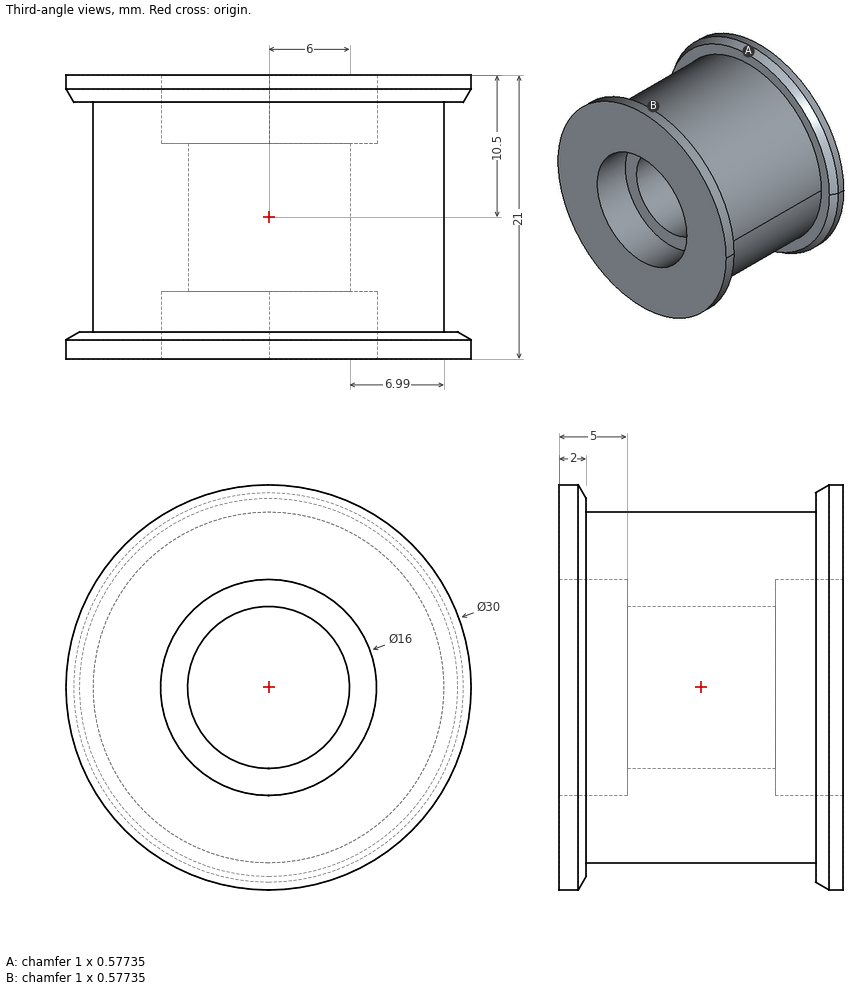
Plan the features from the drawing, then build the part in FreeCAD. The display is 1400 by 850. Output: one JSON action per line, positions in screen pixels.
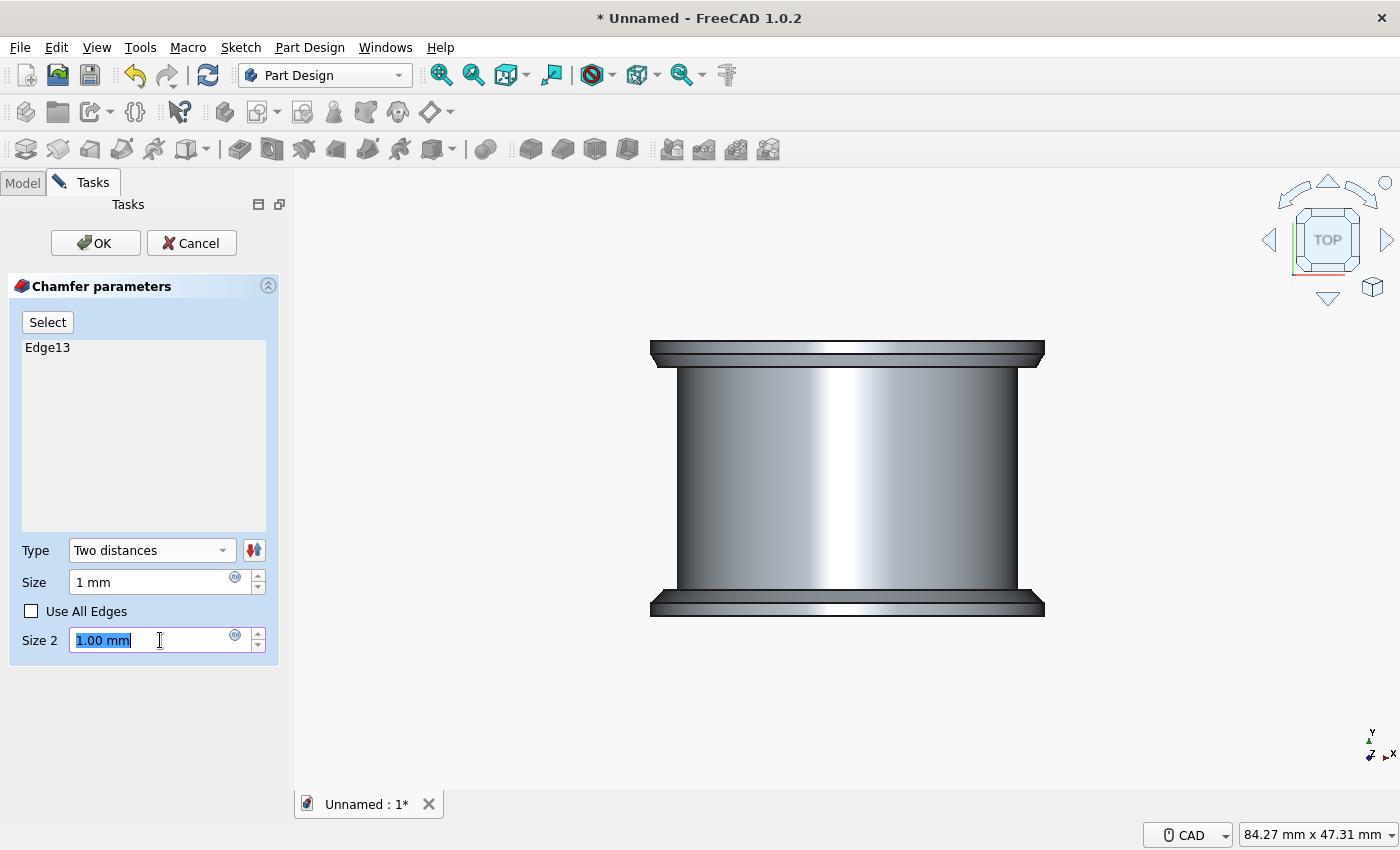
{"action": "type", "text": "0.57735"}
{"action": "key", "text": "Tab"}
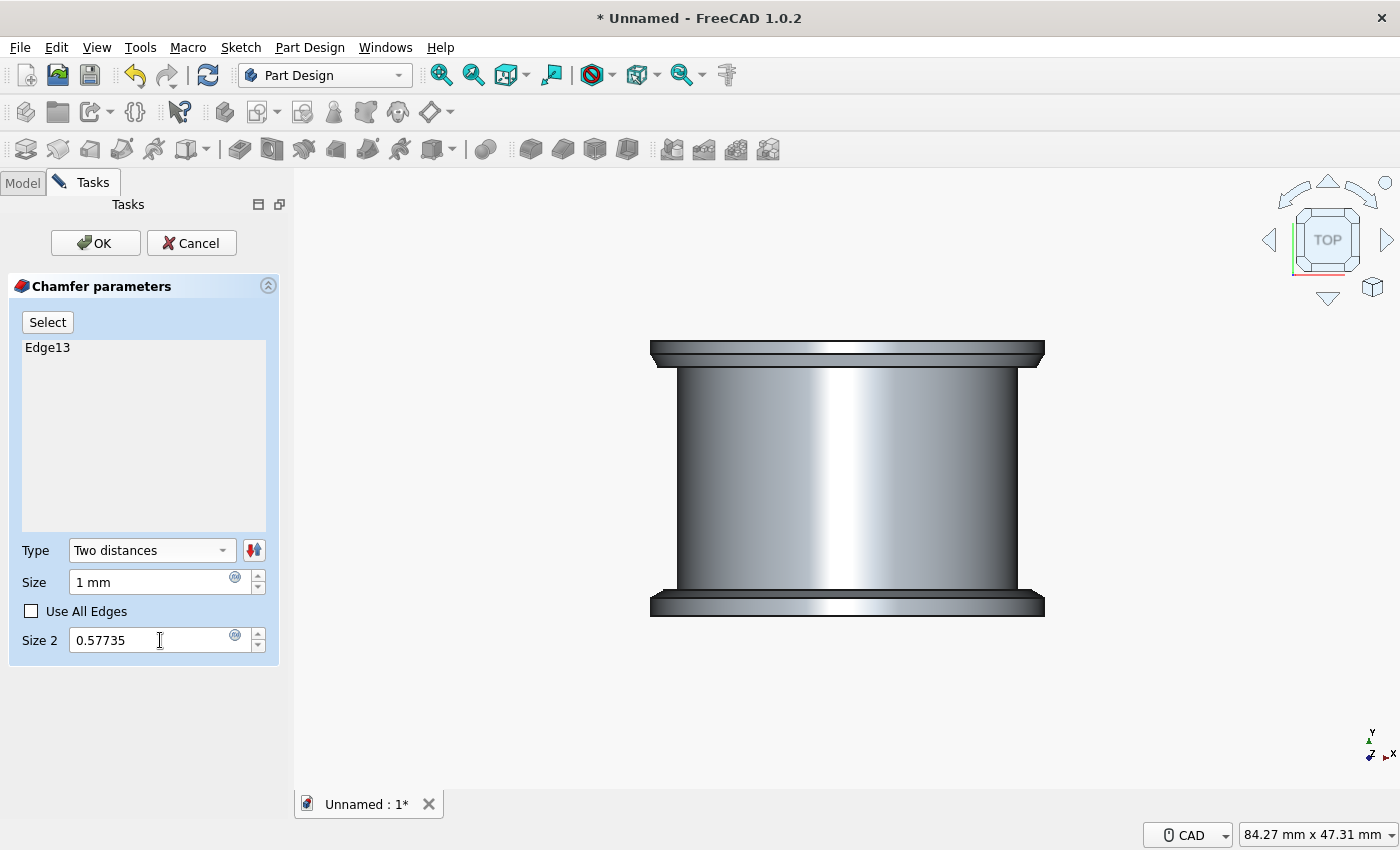
{"action": "left_click", "coordinate": [96, 243]}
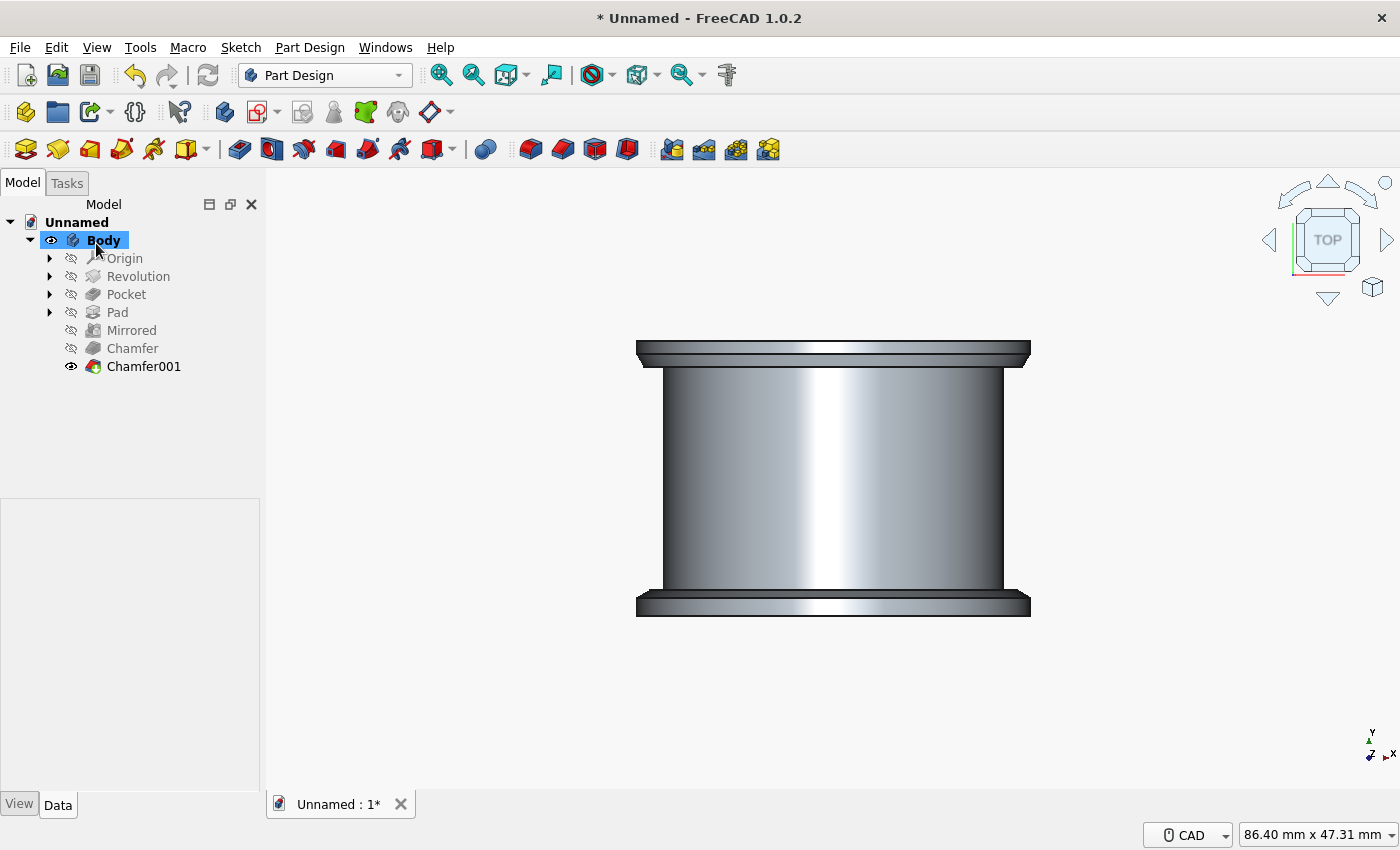
{"action": "key", "text": "0"}